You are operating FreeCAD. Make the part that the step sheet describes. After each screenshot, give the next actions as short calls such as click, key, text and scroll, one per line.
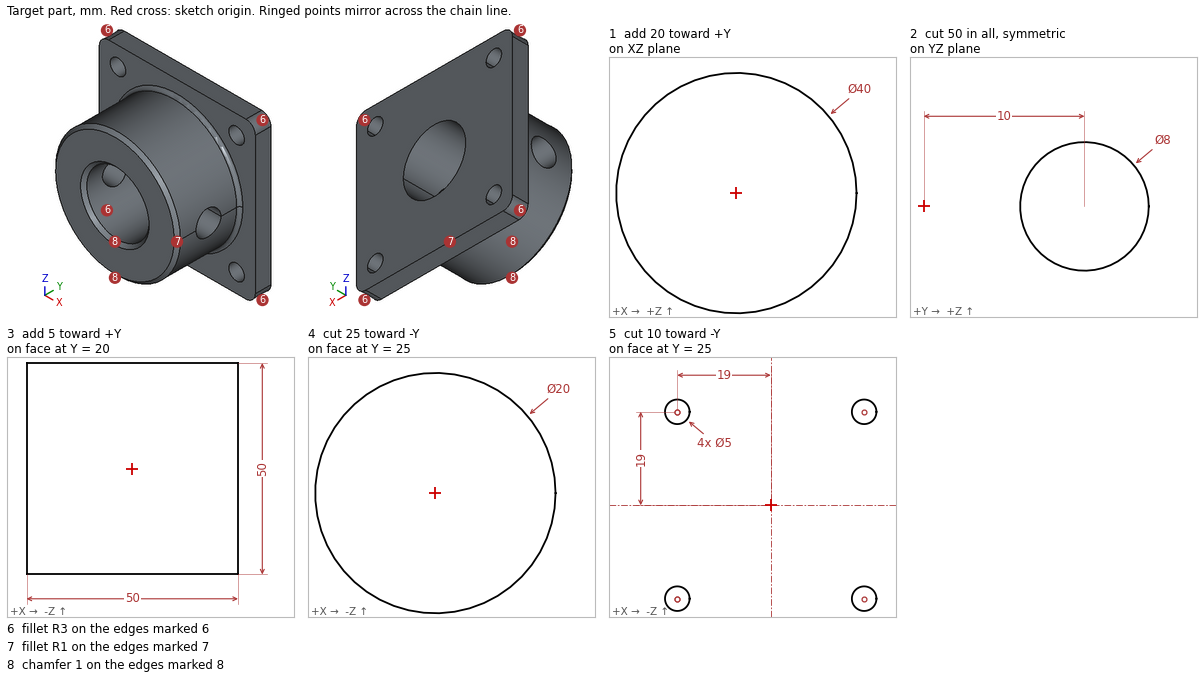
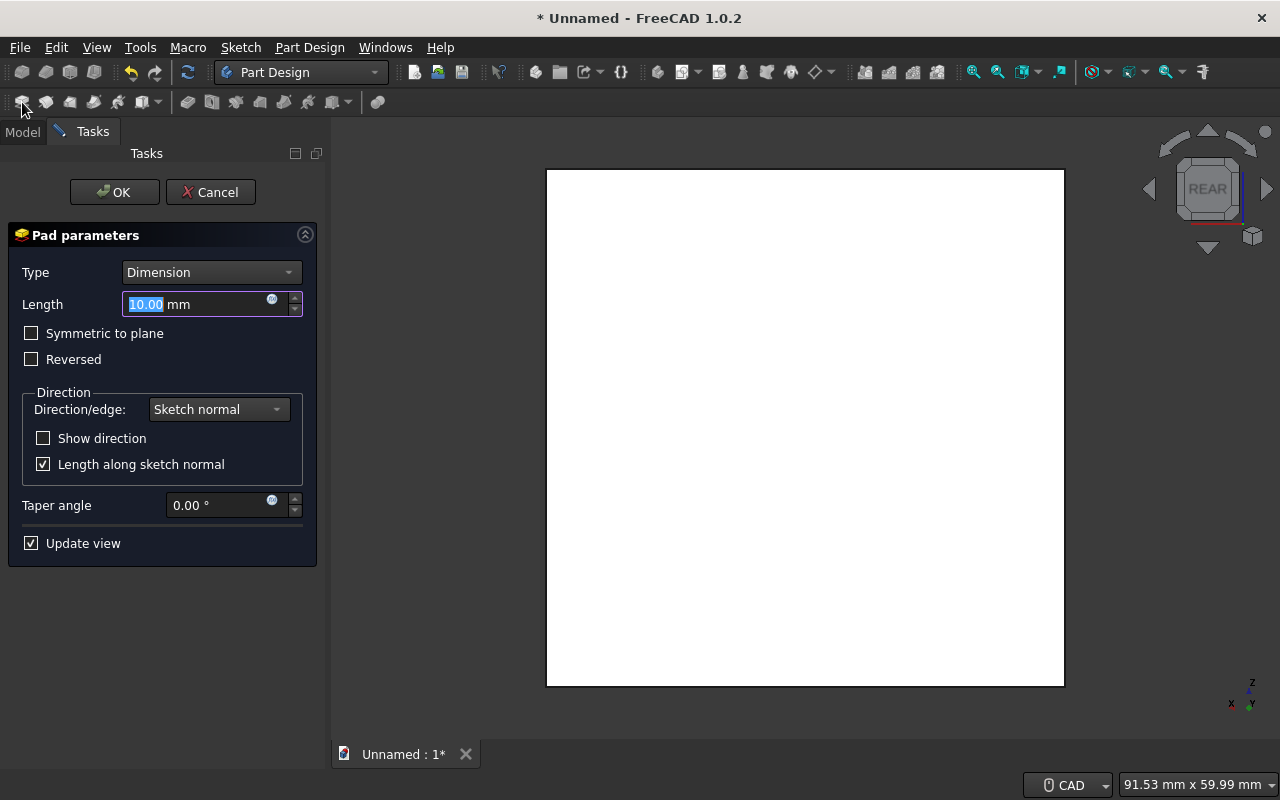
text(5)
key(Tab)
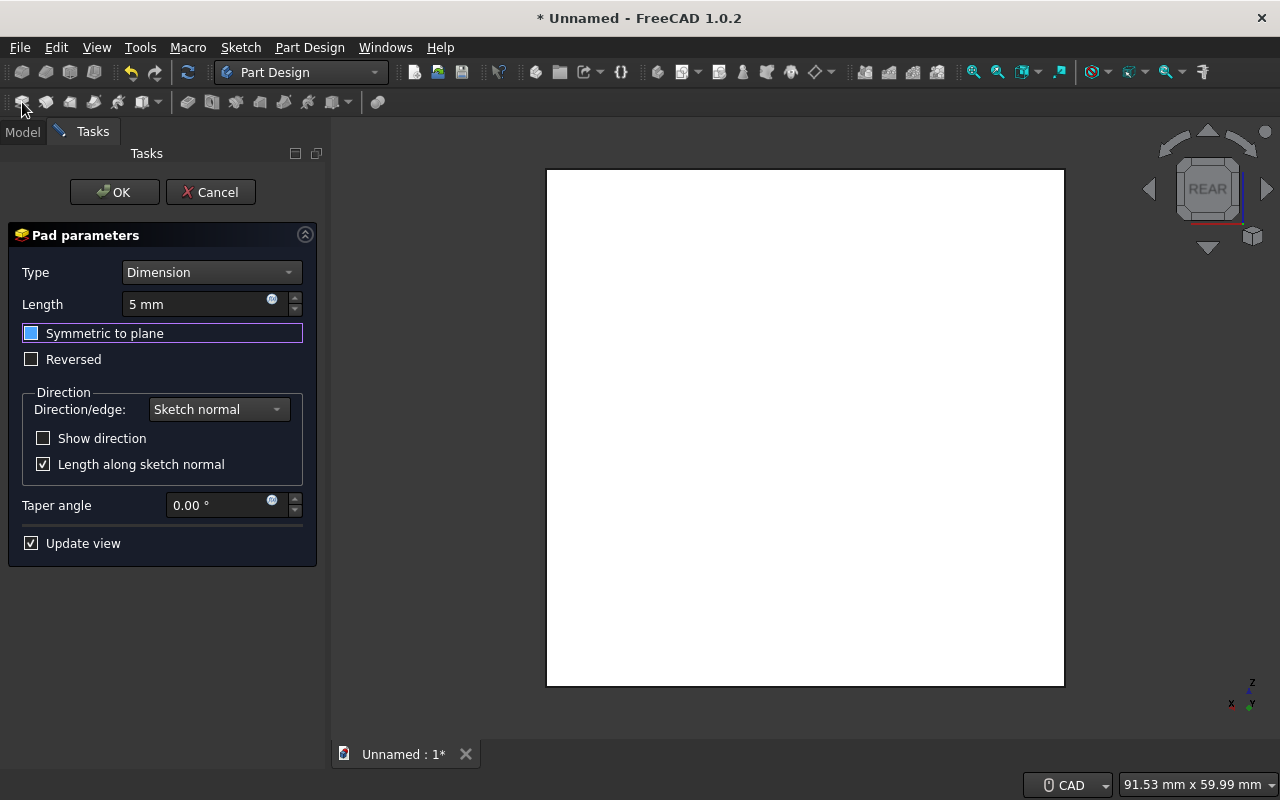
click(115, 192)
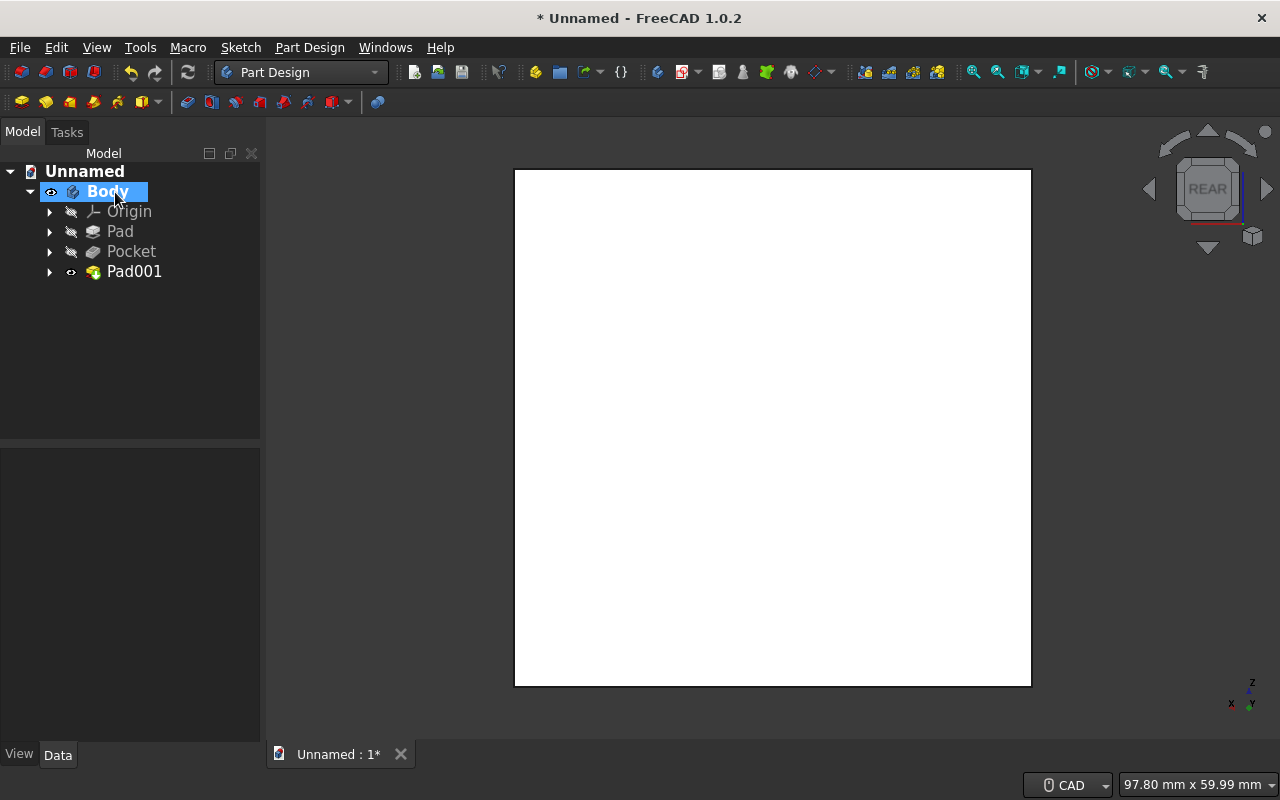
click(773, 427)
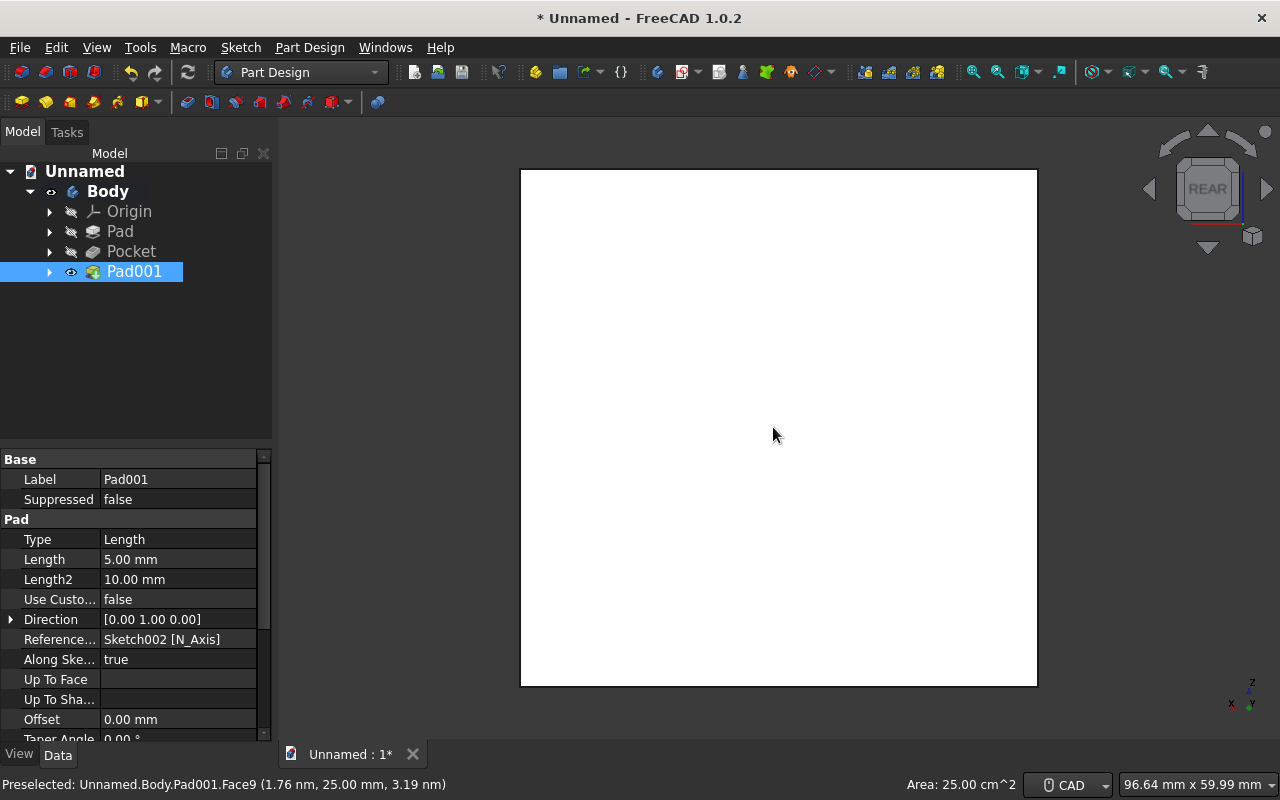
click(682, 72)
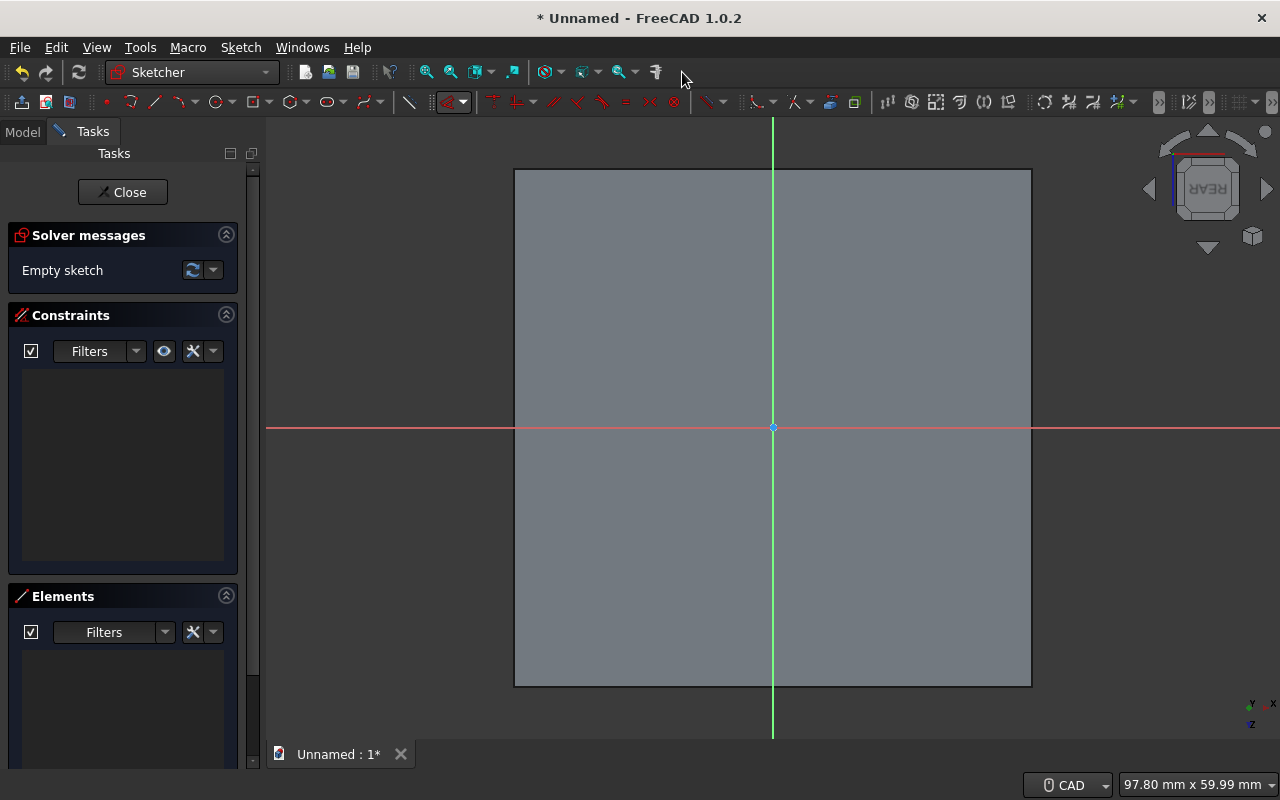
scroll(856, 428, up, 3)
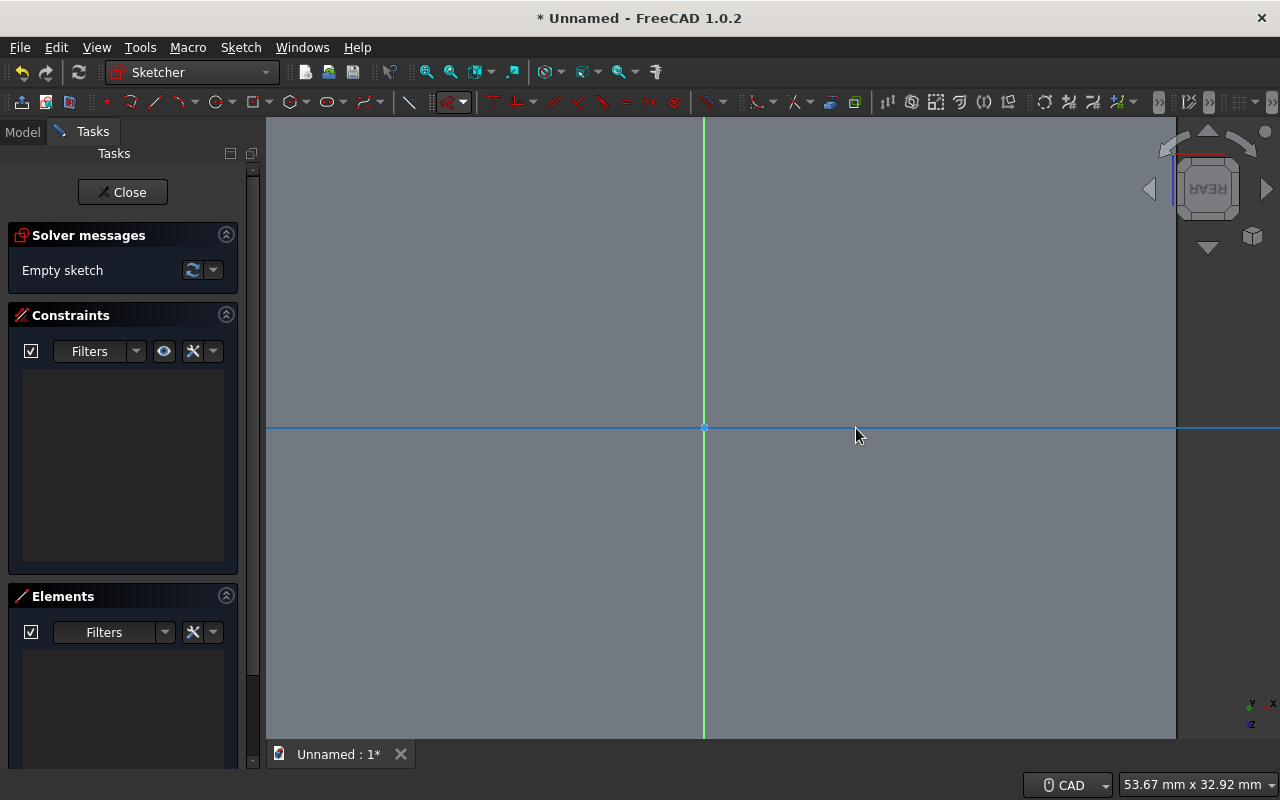
click(216, 102)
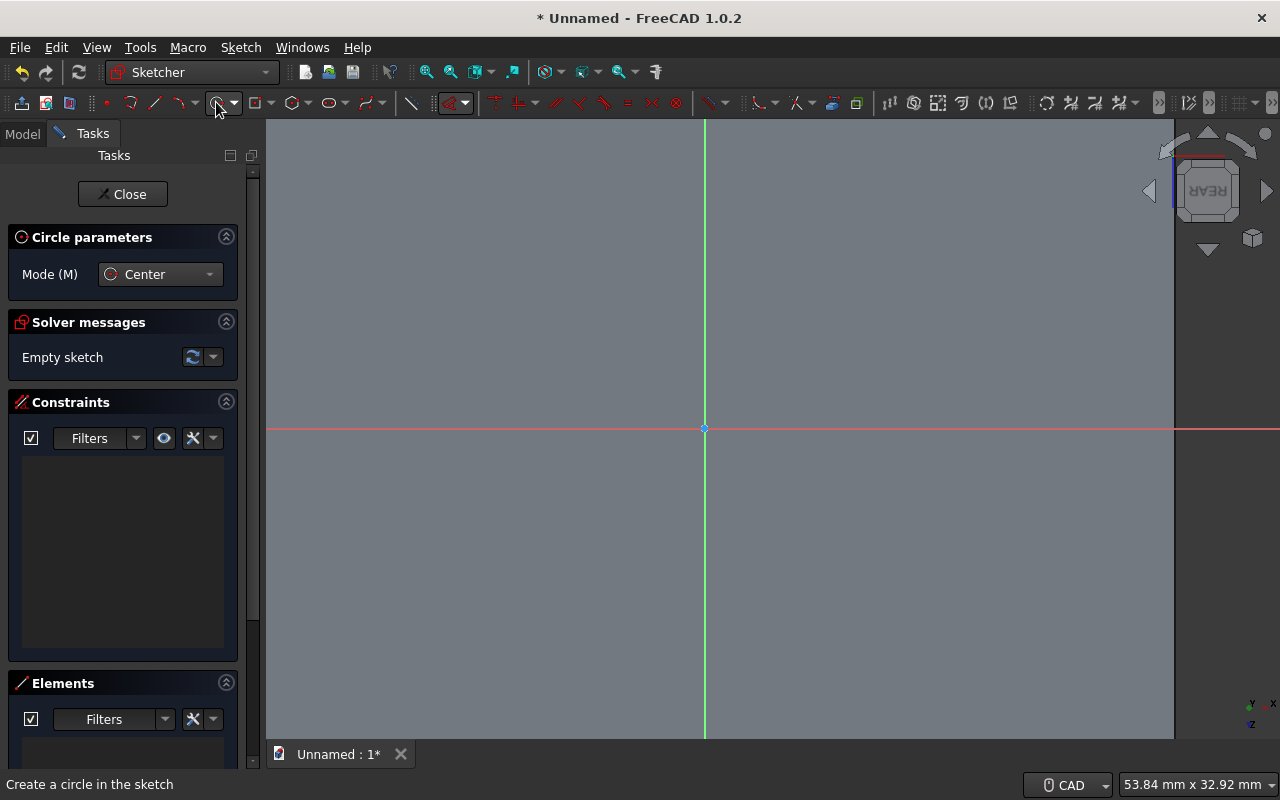
click(705, 429)
click(838, 295)
key(Escape)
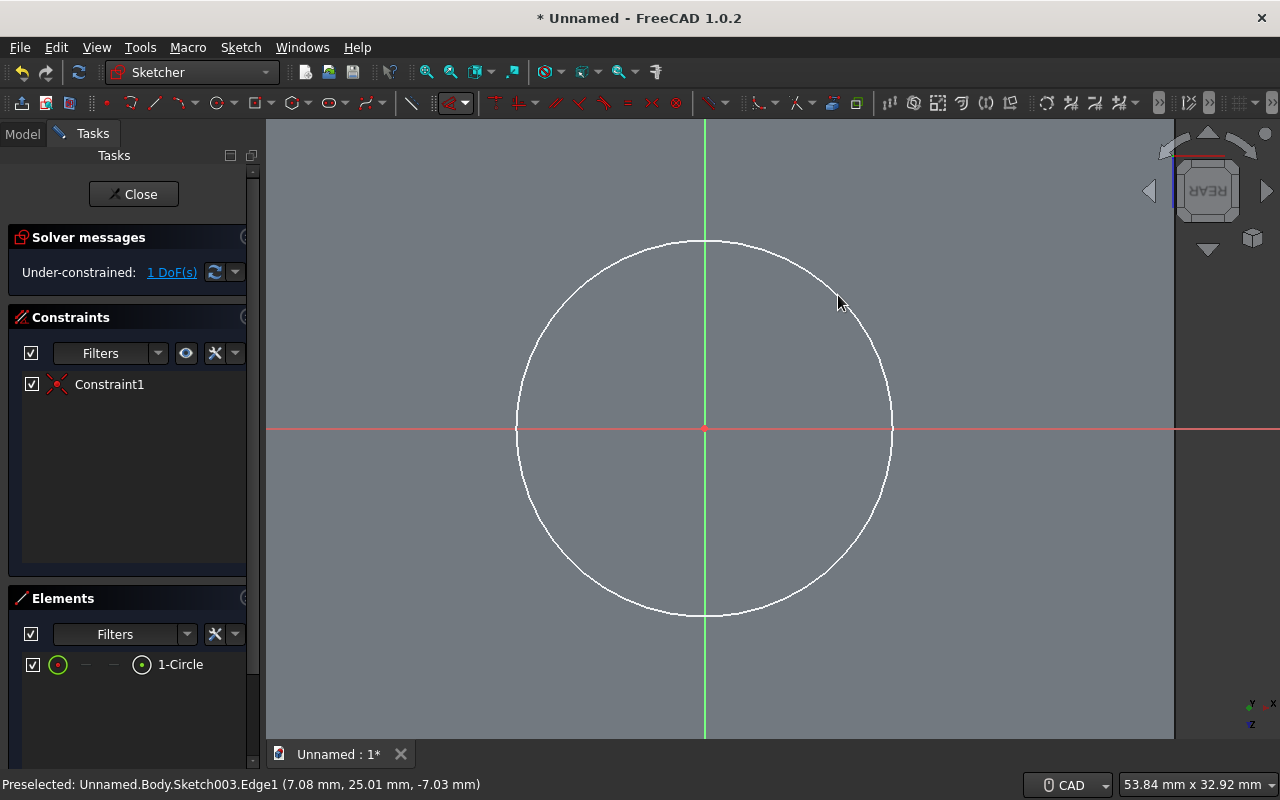
click(837, 295)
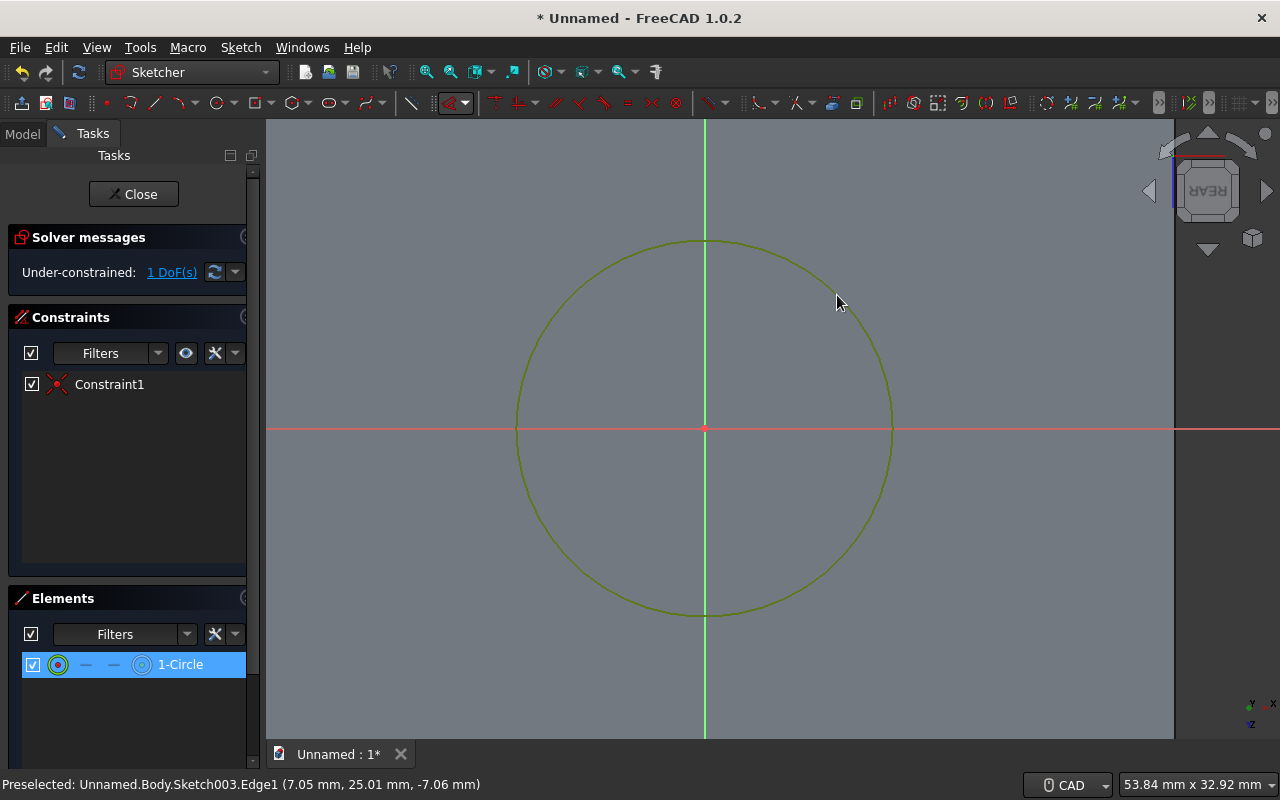
key(k)
key(o)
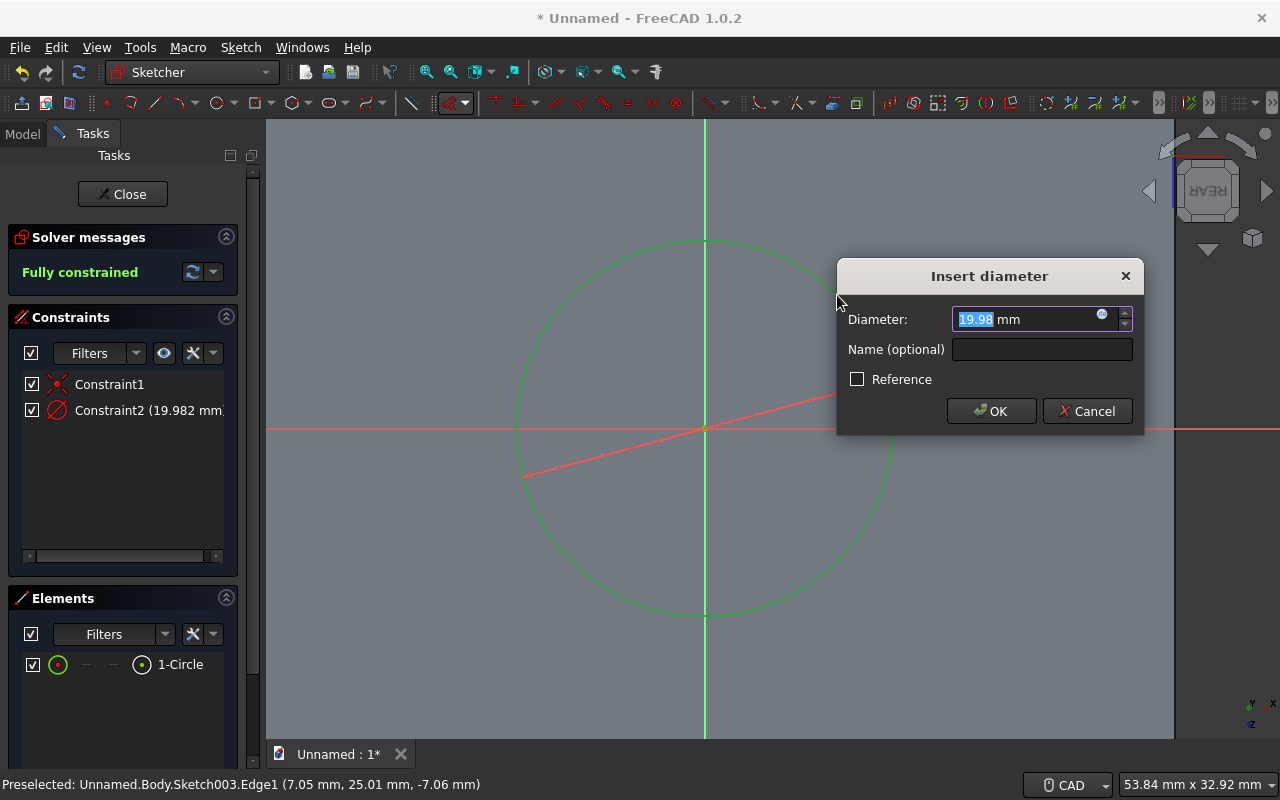
text(20)
key(Return)